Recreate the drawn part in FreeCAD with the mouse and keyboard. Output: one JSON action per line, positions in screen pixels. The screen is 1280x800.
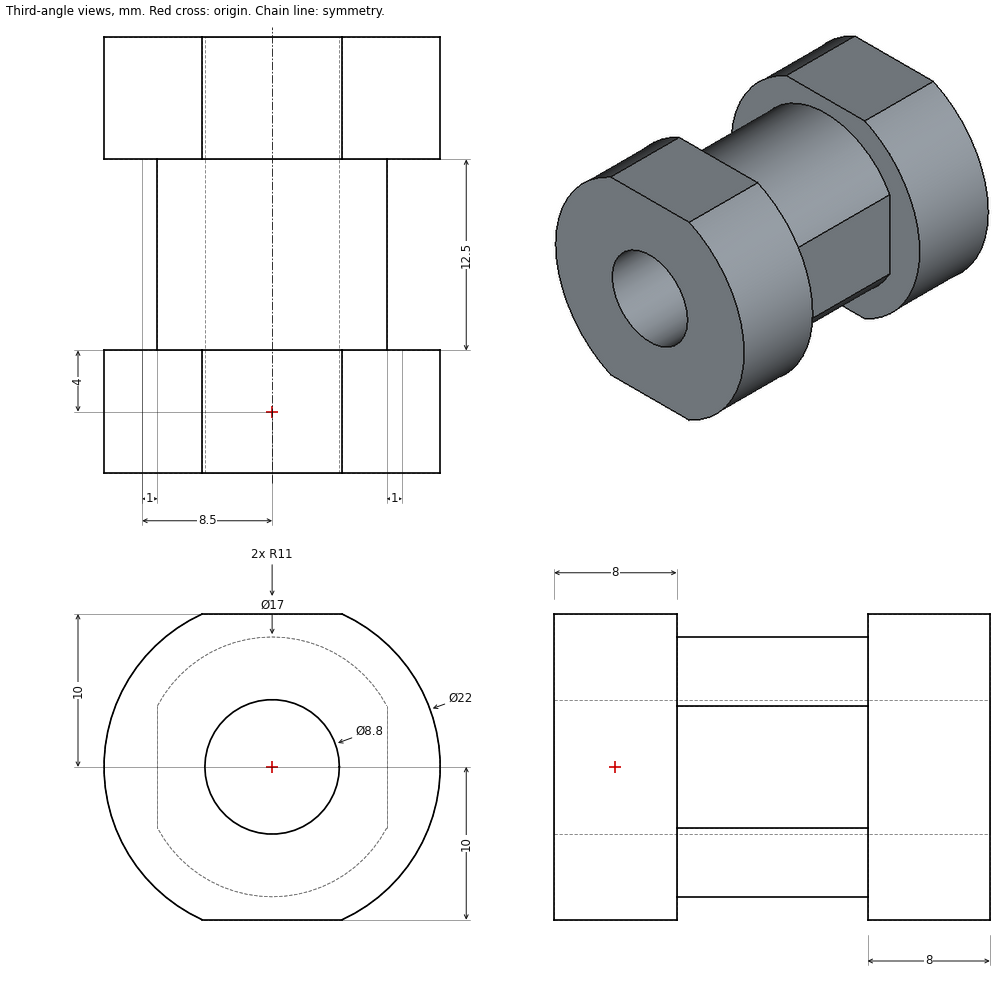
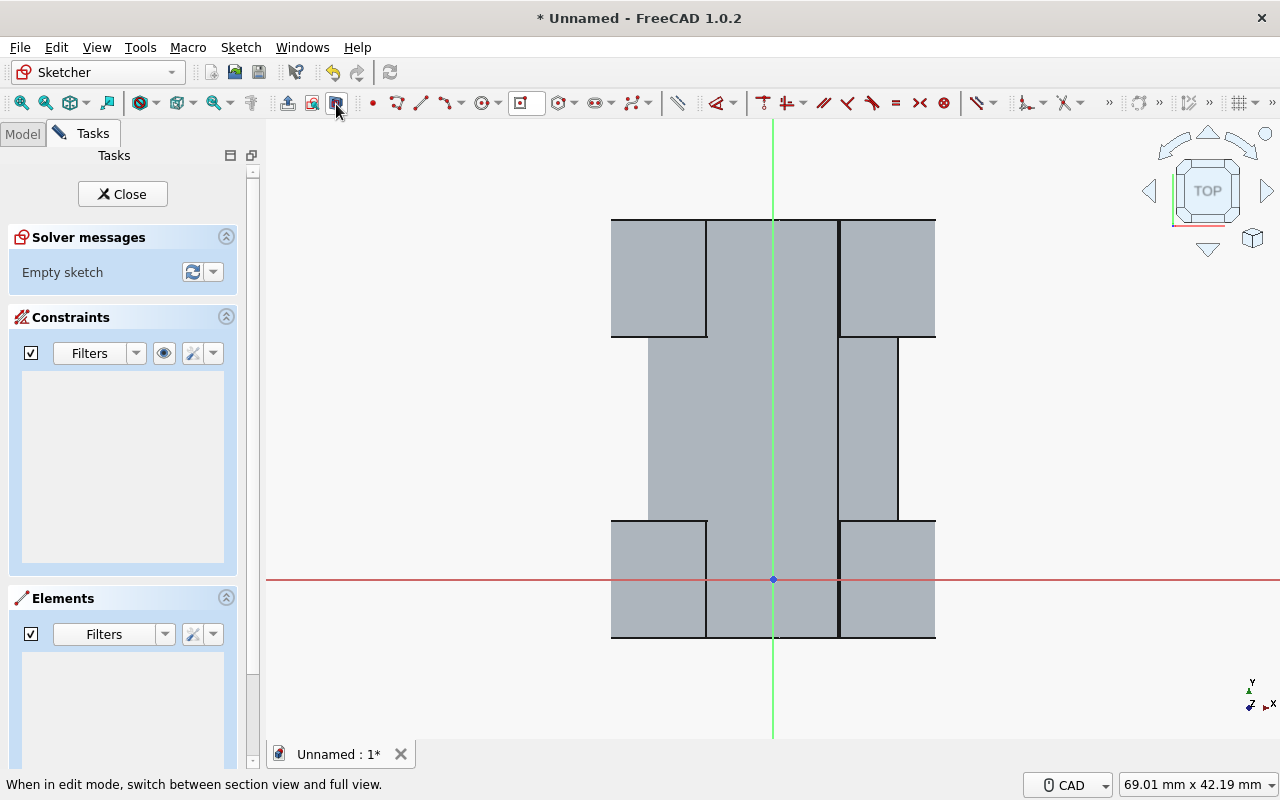
{"action": "scroll", "coordinate": [912, 518], "scroll_direction": "up", "scroll_amount": 2}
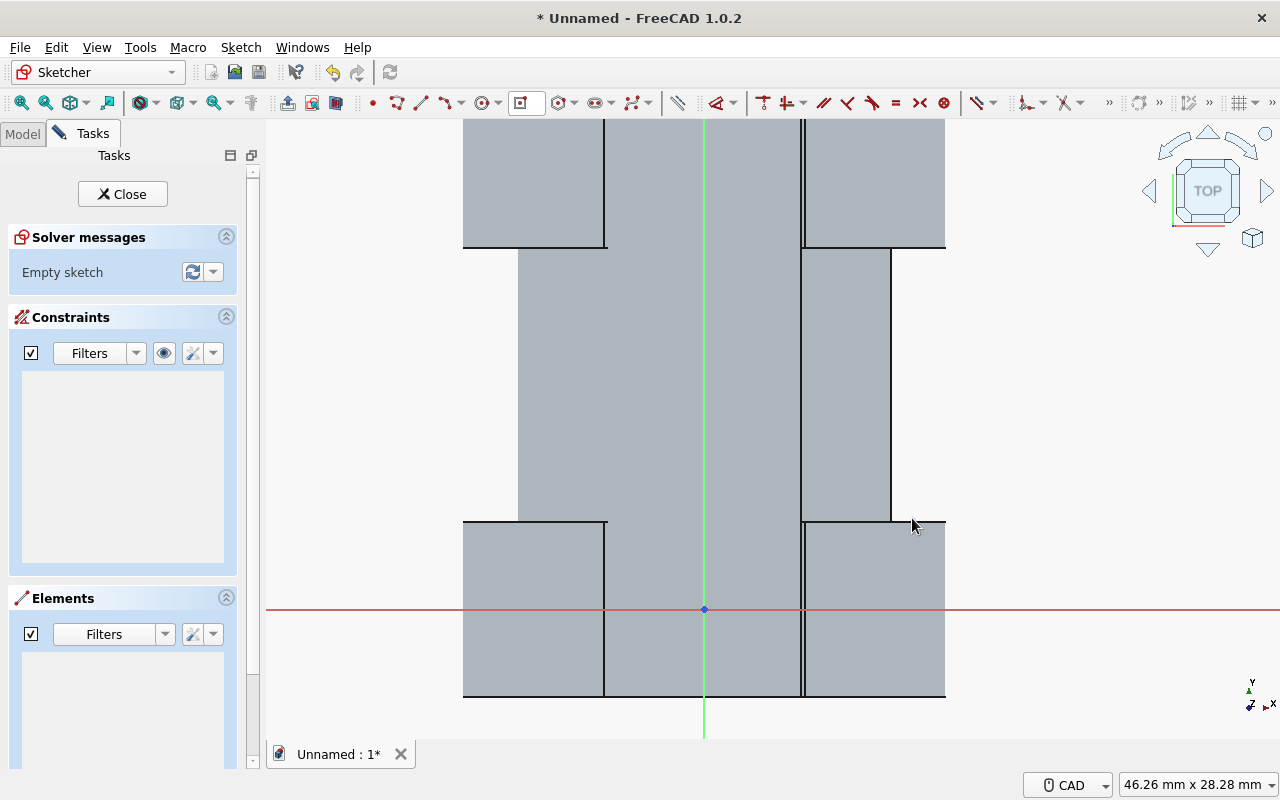
{"action": "key", "text": "g r"}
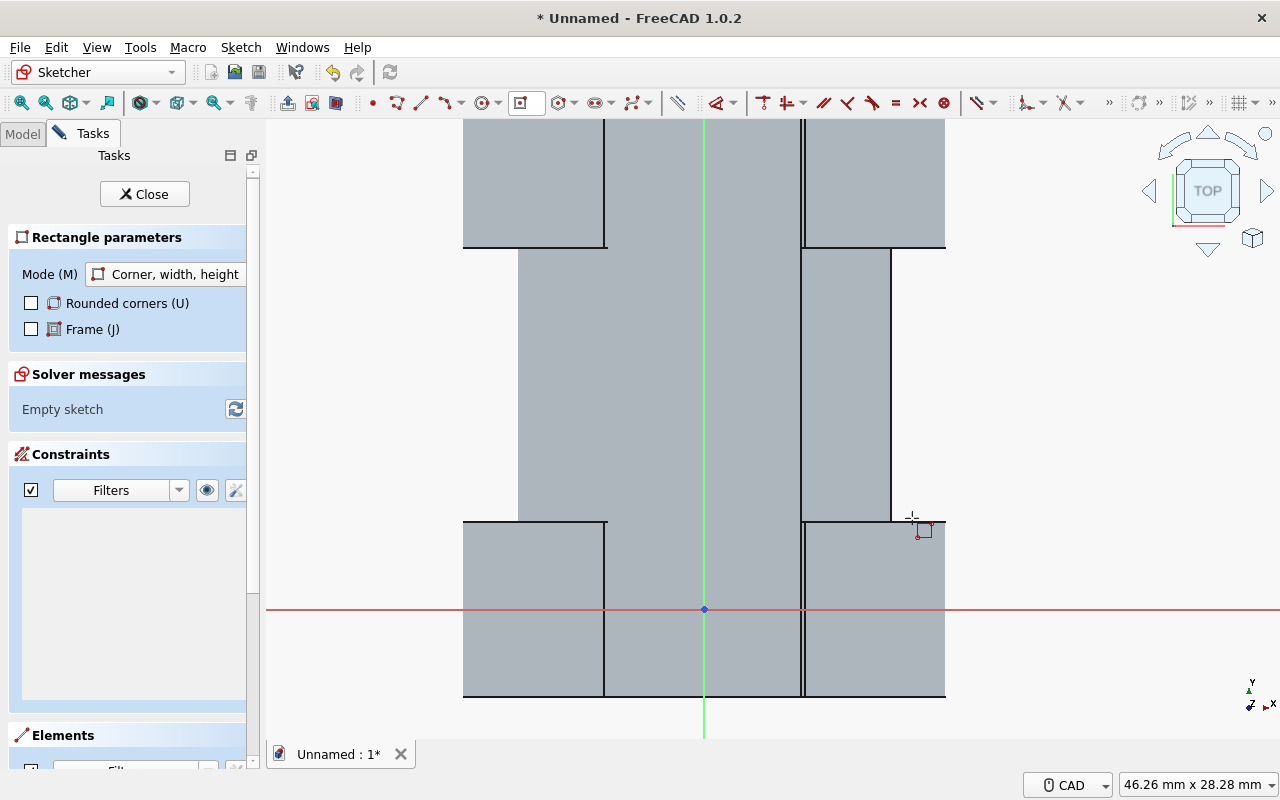
{"action": "left_click", "coordinate": [518, 248]}
{"action": "mouse_move", "coordinate": [540, 522]}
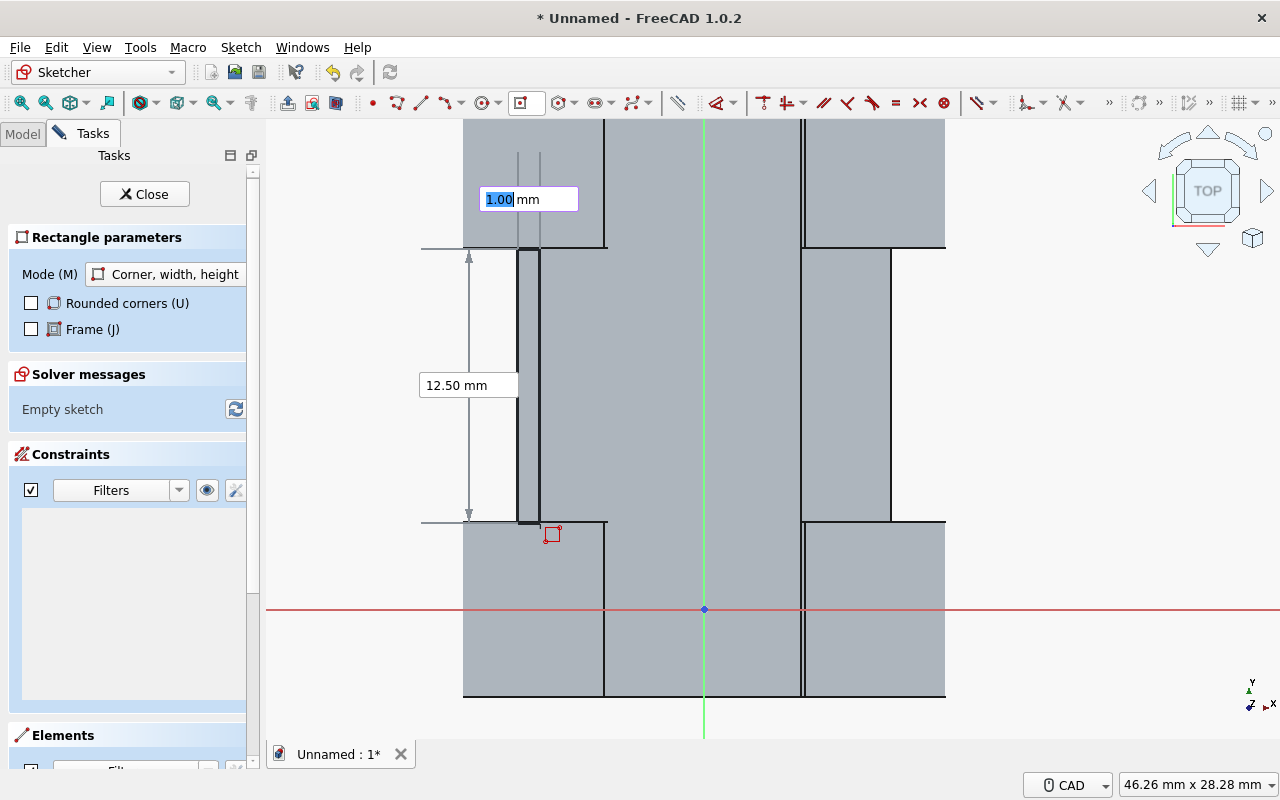
{"action": "type", "text": "1"}
{"action": "key", "text": "Tab"}
{"action": "type", "text": "12.5"}
{"action": "key", "text": "Return"}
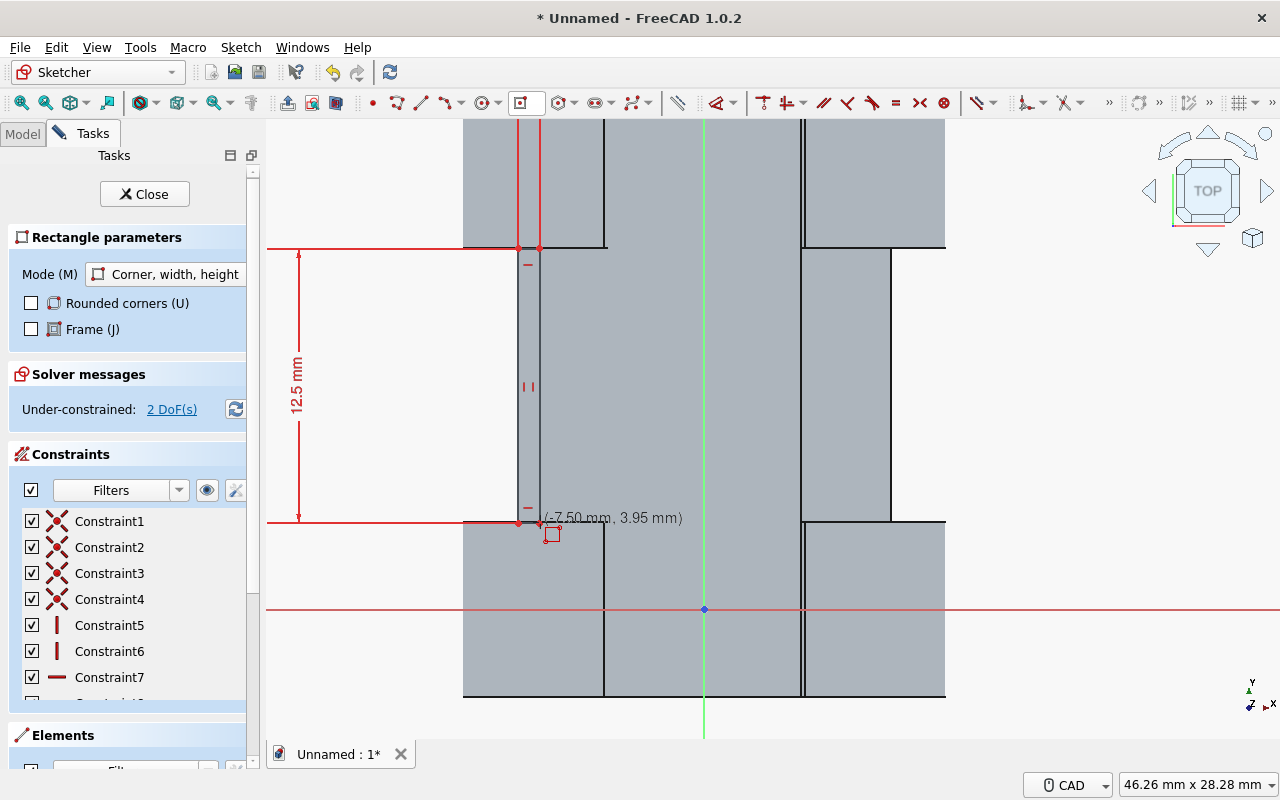
{"action": "left_click", "coordinate": [869, 248]}
{"action": "mouse_move", "coordinate": [891, 522]}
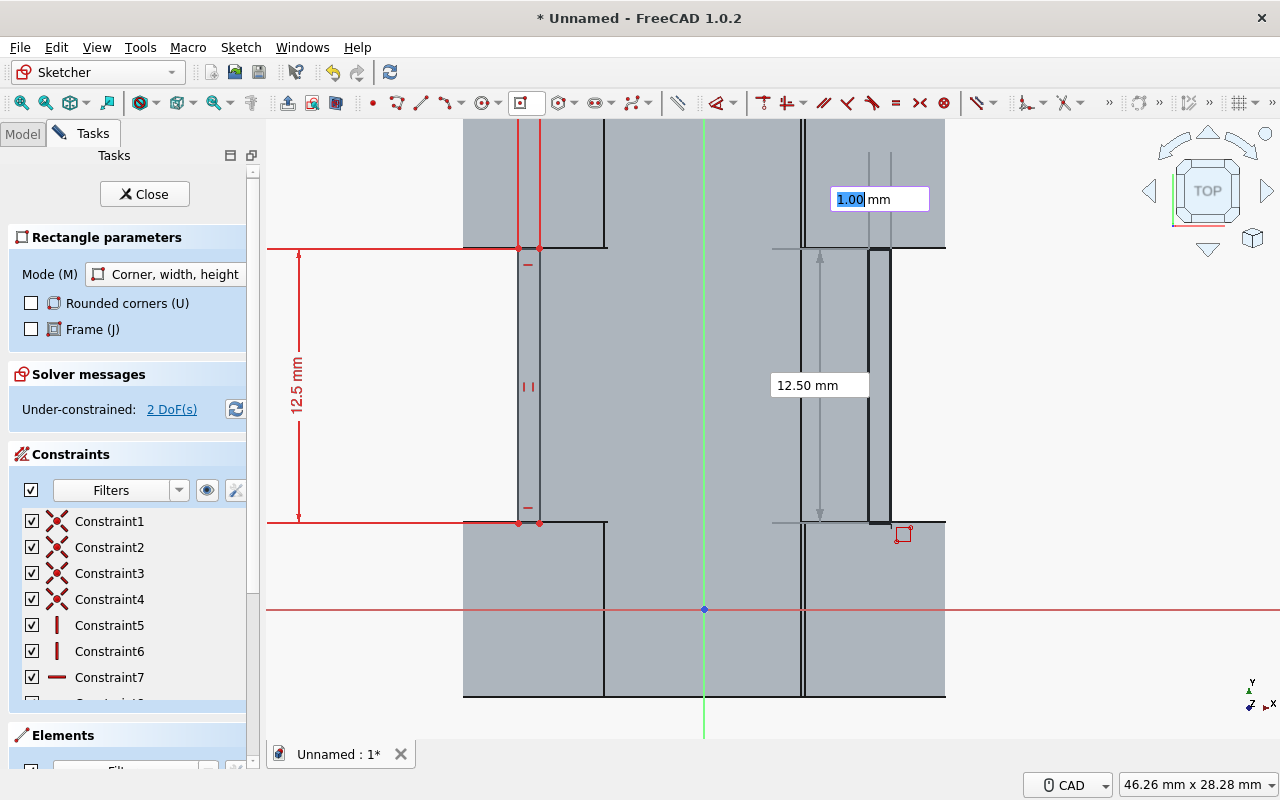
{"action": "type", "text": "1"}
{"action": "key", "text": "Tab"}
{"action": "type", "text": "12.5"}
{"action": "key", "text": "Return"}
{"action": "key", "text": "Escape"}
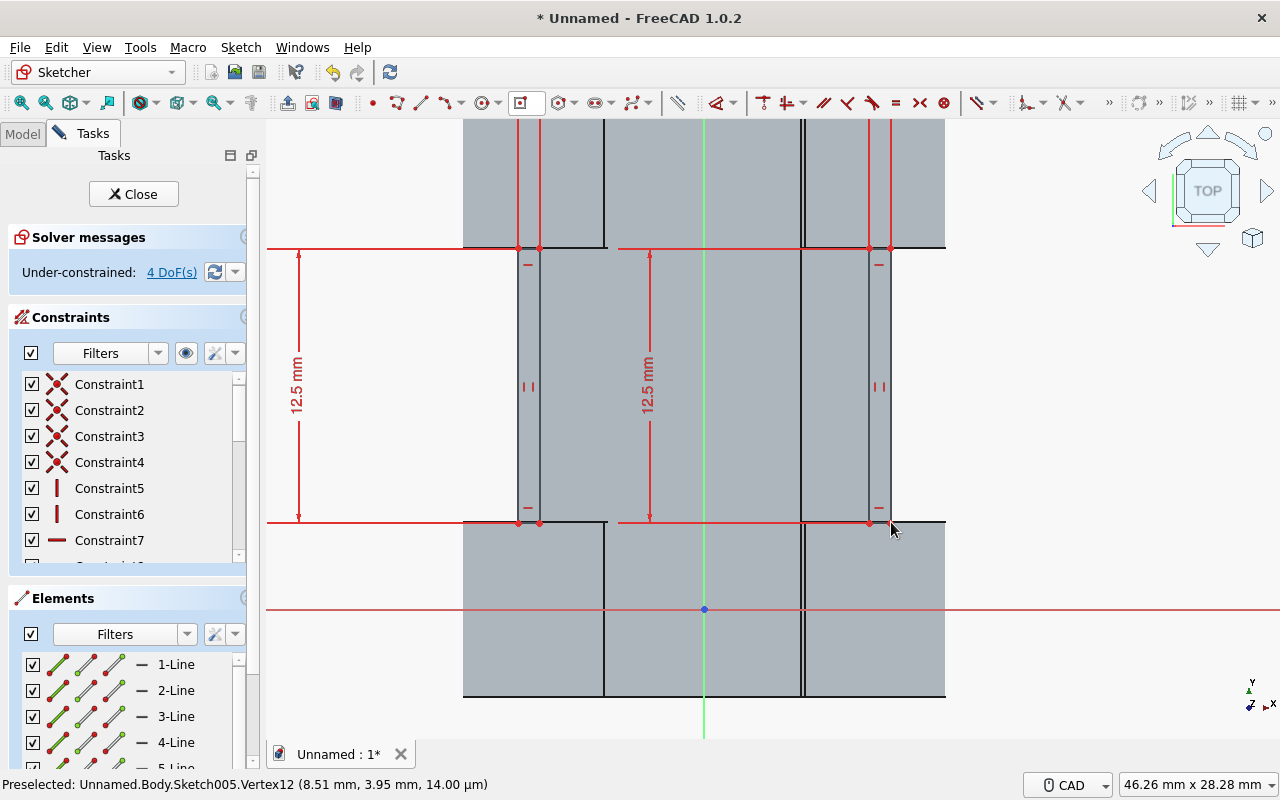
{"action": "left_click", "coordinate": [540, 249]}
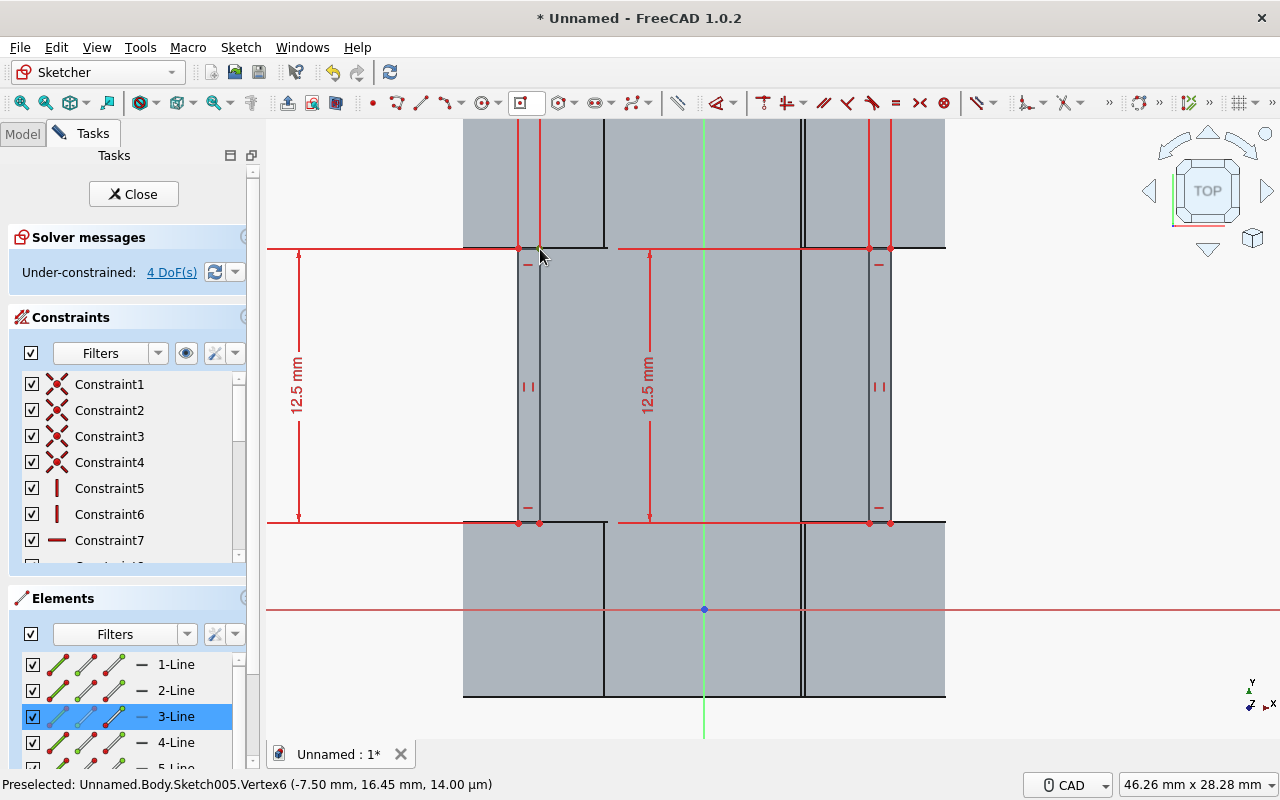
{"action": "left_click", "coordinate": [869, 249]}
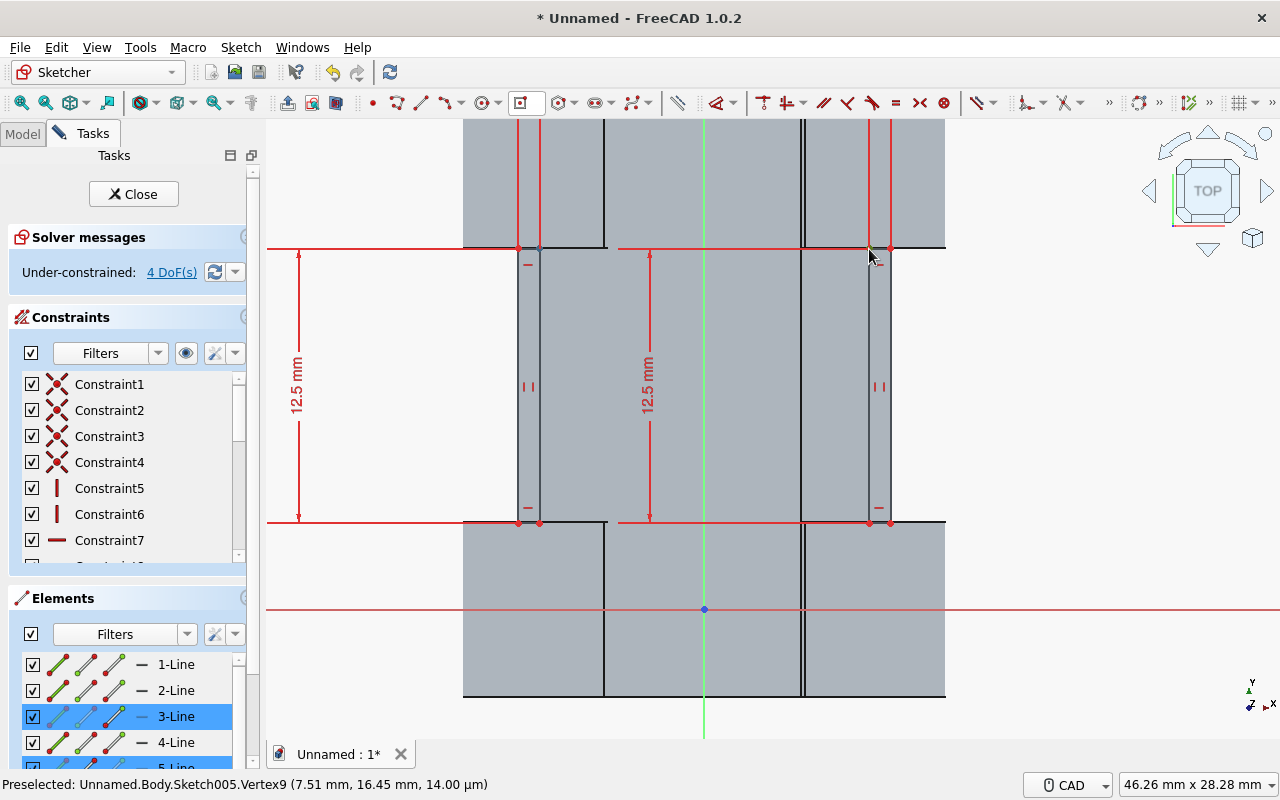
{"action": "left_click", "coordinate": [704, 671]}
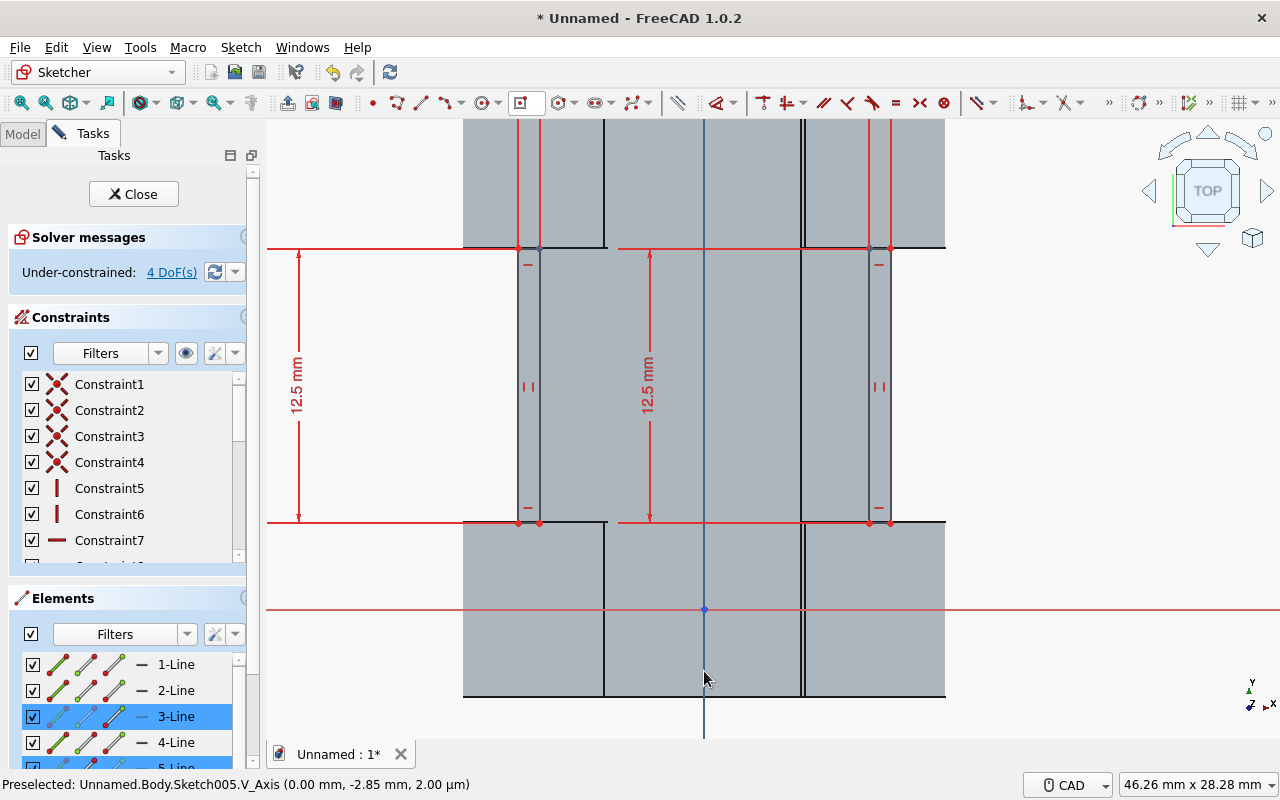
{"action": "left_click", "coordinate": [920, 104]}